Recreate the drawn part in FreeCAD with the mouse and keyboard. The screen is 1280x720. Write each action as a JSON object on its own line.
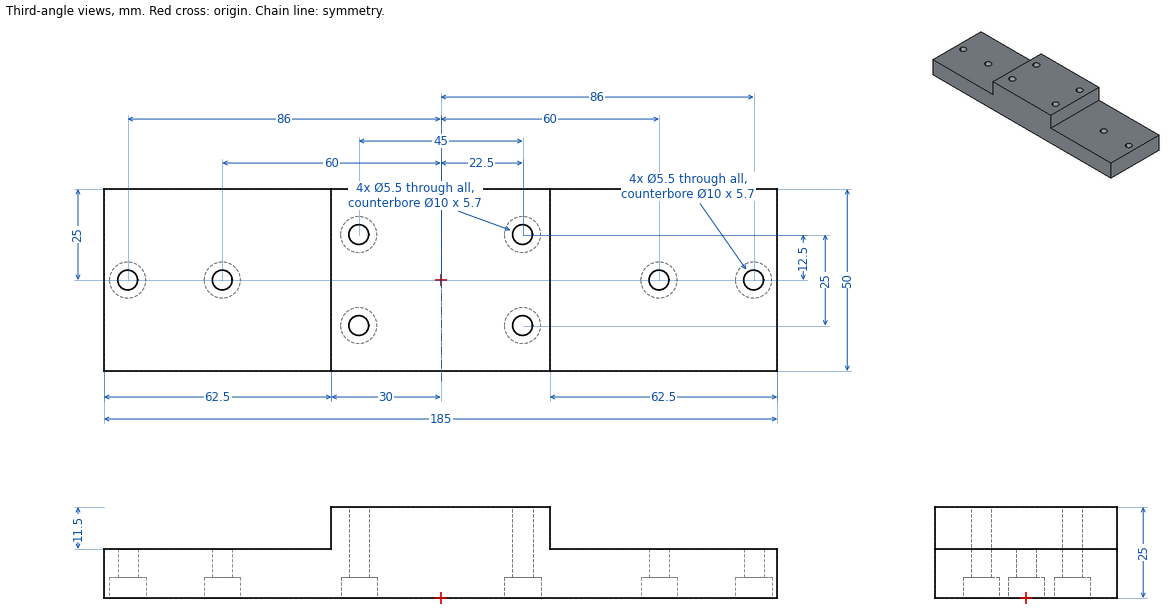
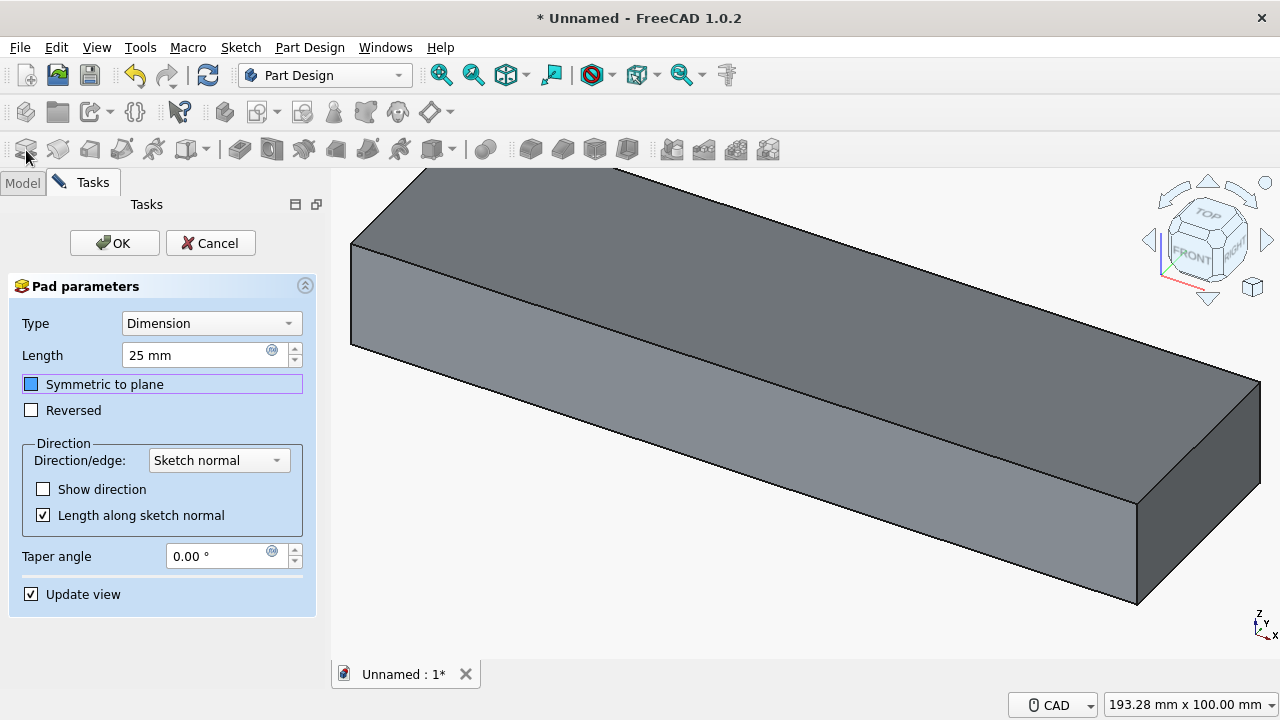
{"action": "left_click", "coordinate": [115, 243]}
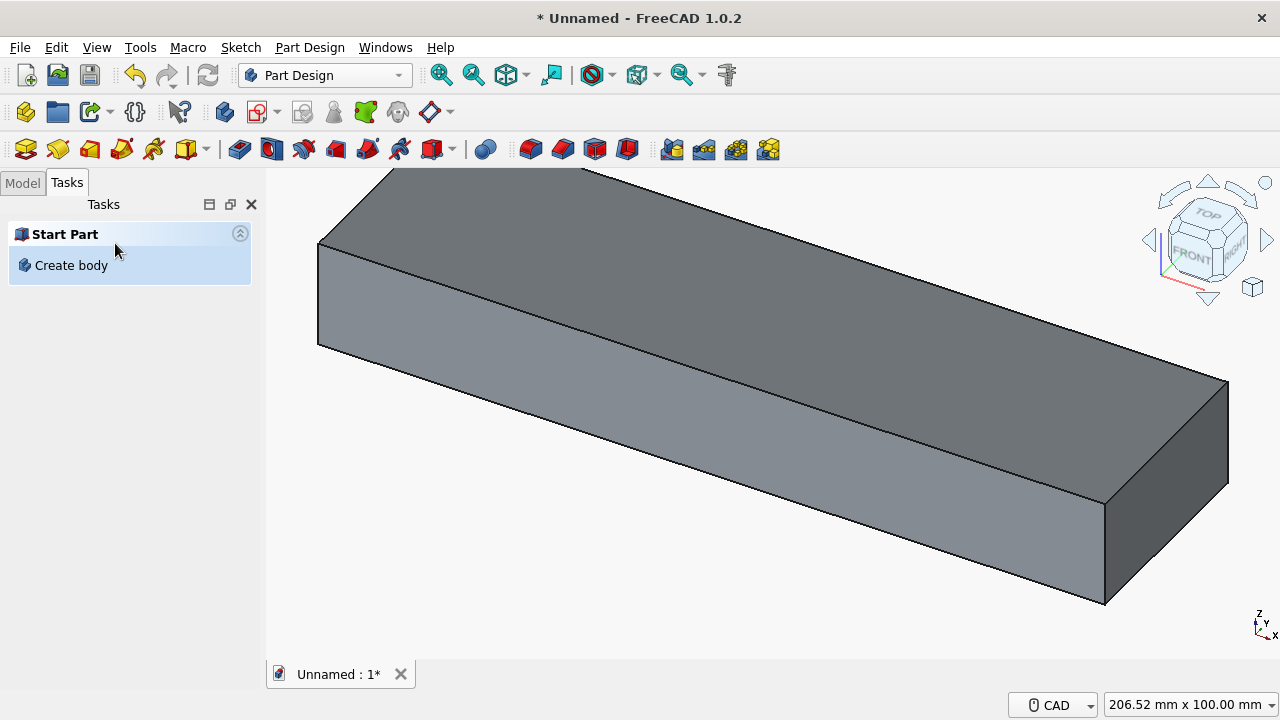
{"action": "key", "text": "v f"}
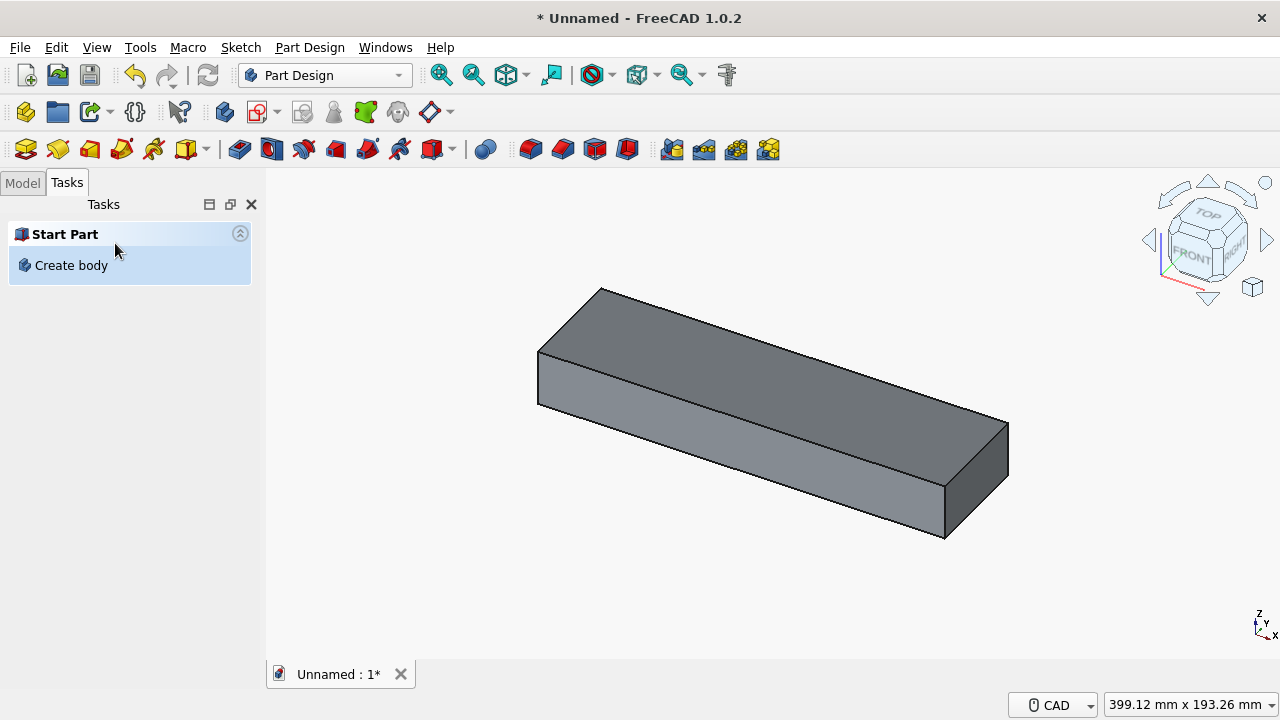
{"action": "left_click", "coordinate": [889, 425]}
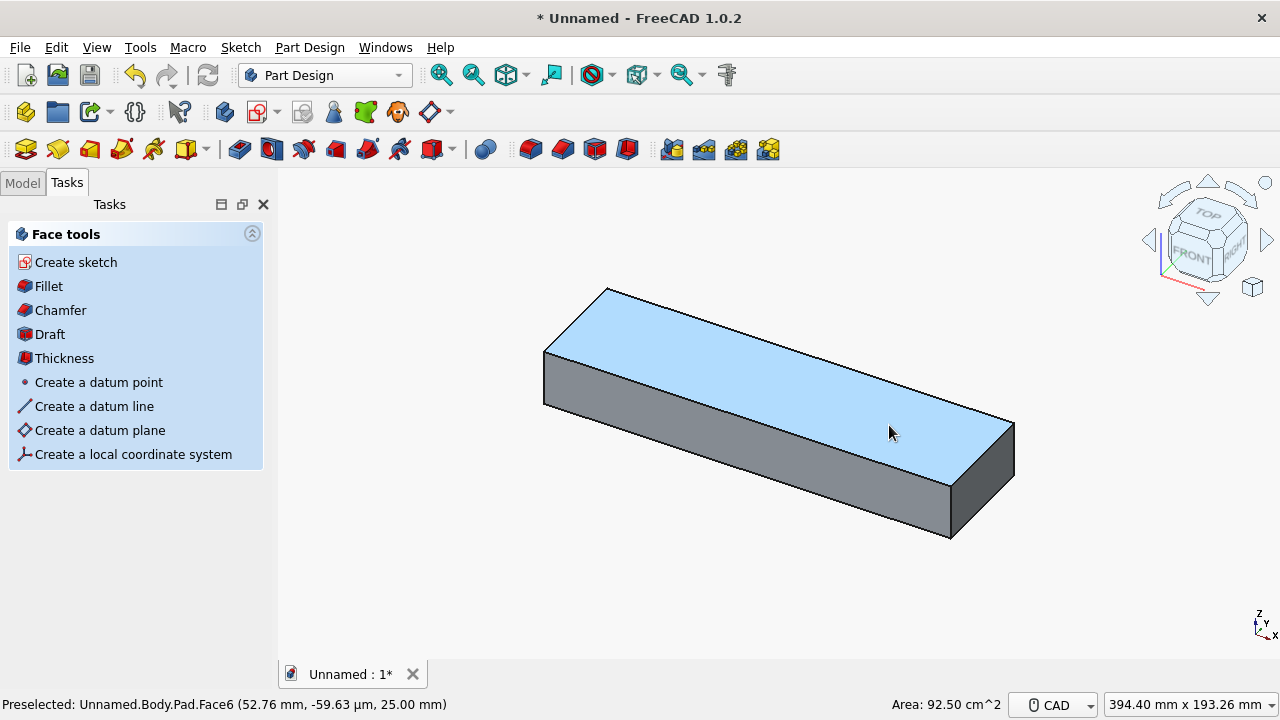
{"action": "left_click", "coordinate": [258, 112]}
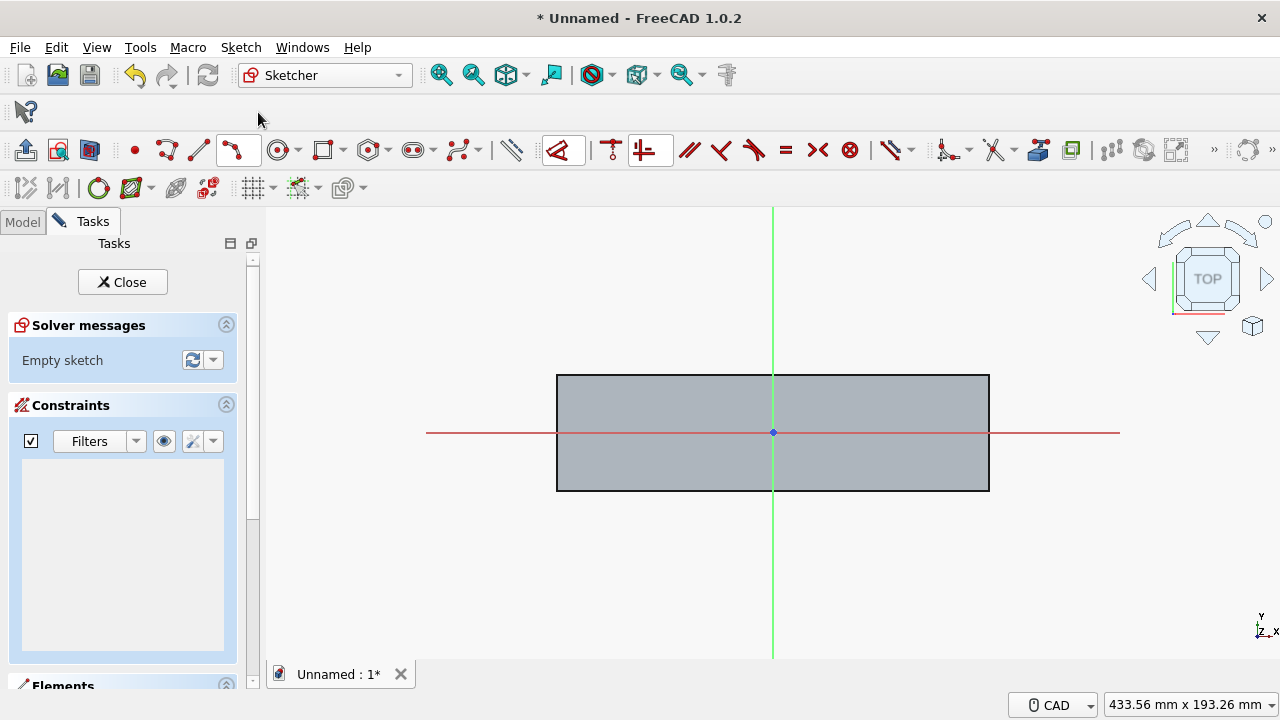
{"action": "key", "text": "g r"}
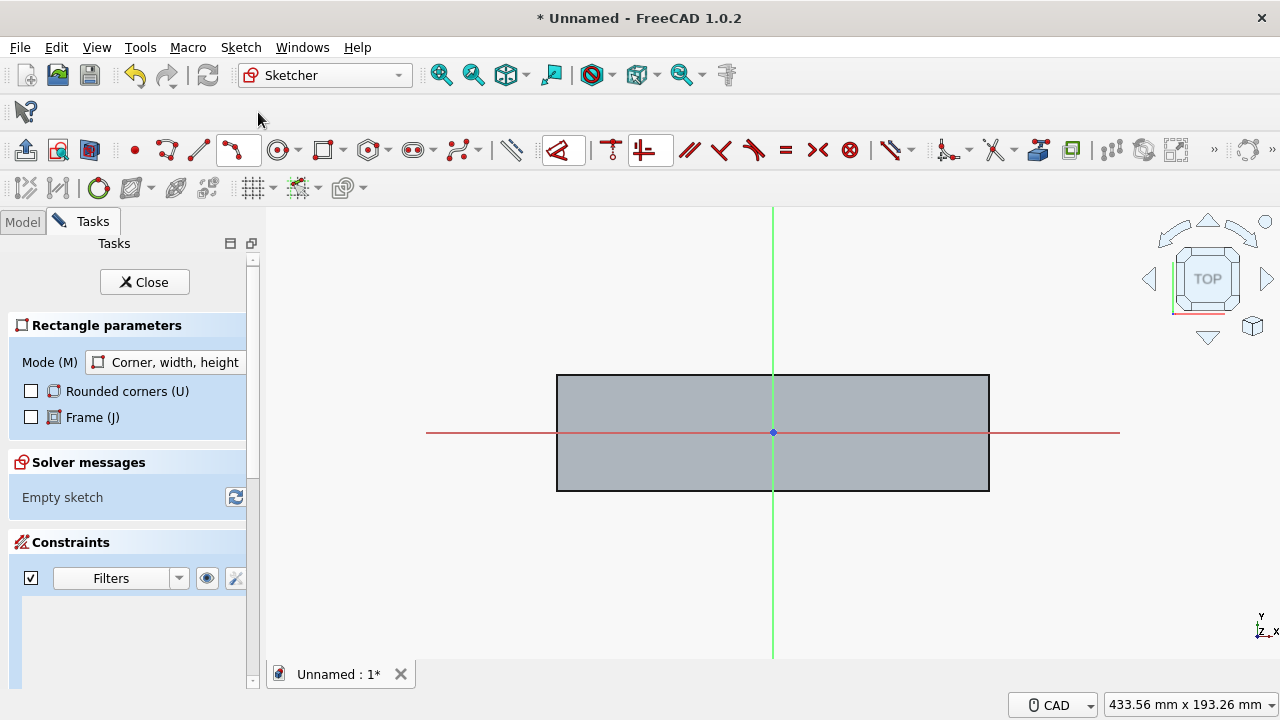
{"action": "left_click", "coordinate": [557, 375]}
{"action": "mouse_move", "coordinate": [703, 491]}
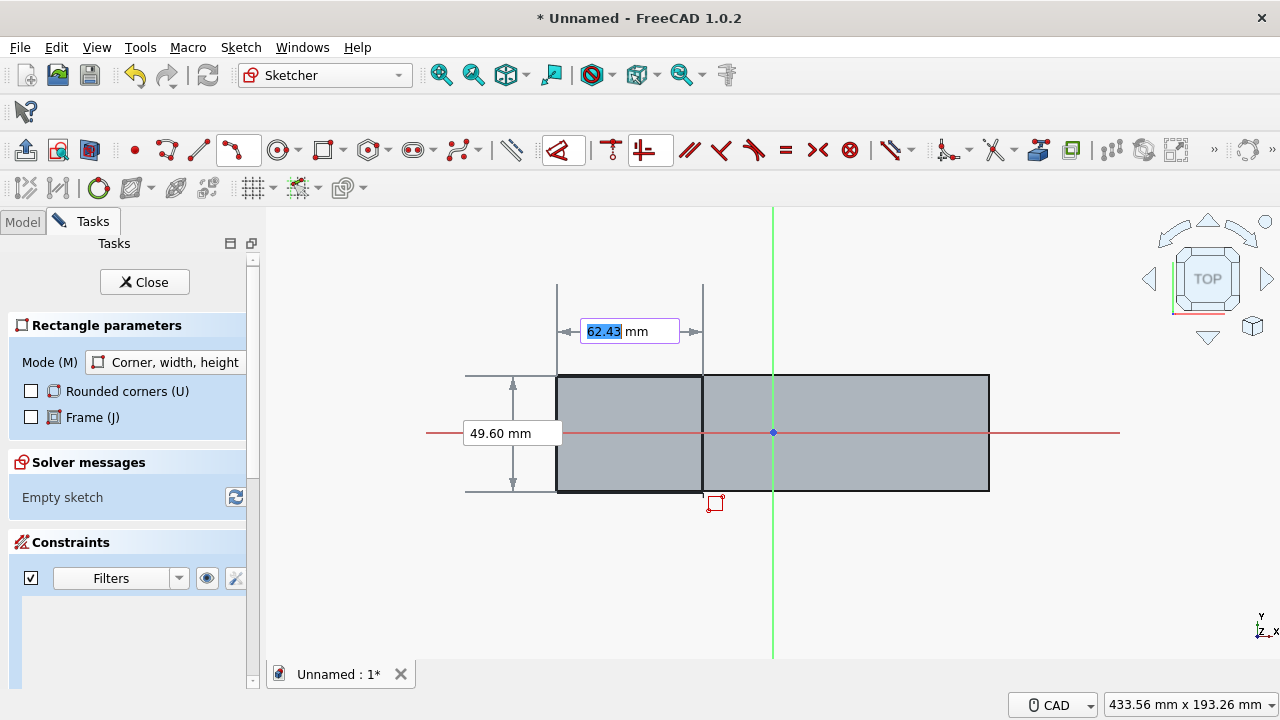
{"action": "type", "text": "62.5"}
{"action": "key", "text": "Tab"}
{"action": "type", "text": "50"}
{"action": "key", "text": "Return"}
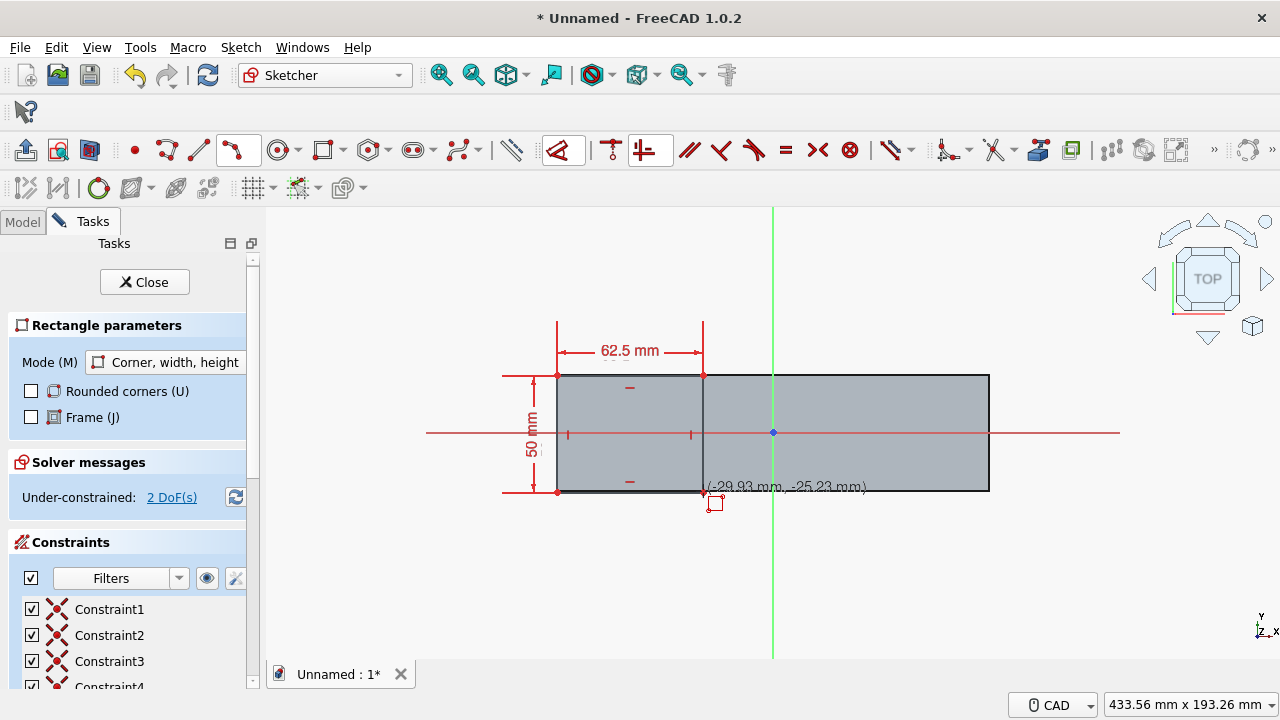
{"action": "left_click", "coordinate": [843, 375]}
{"action": "mouse_move", "coordinate": [989, 491]}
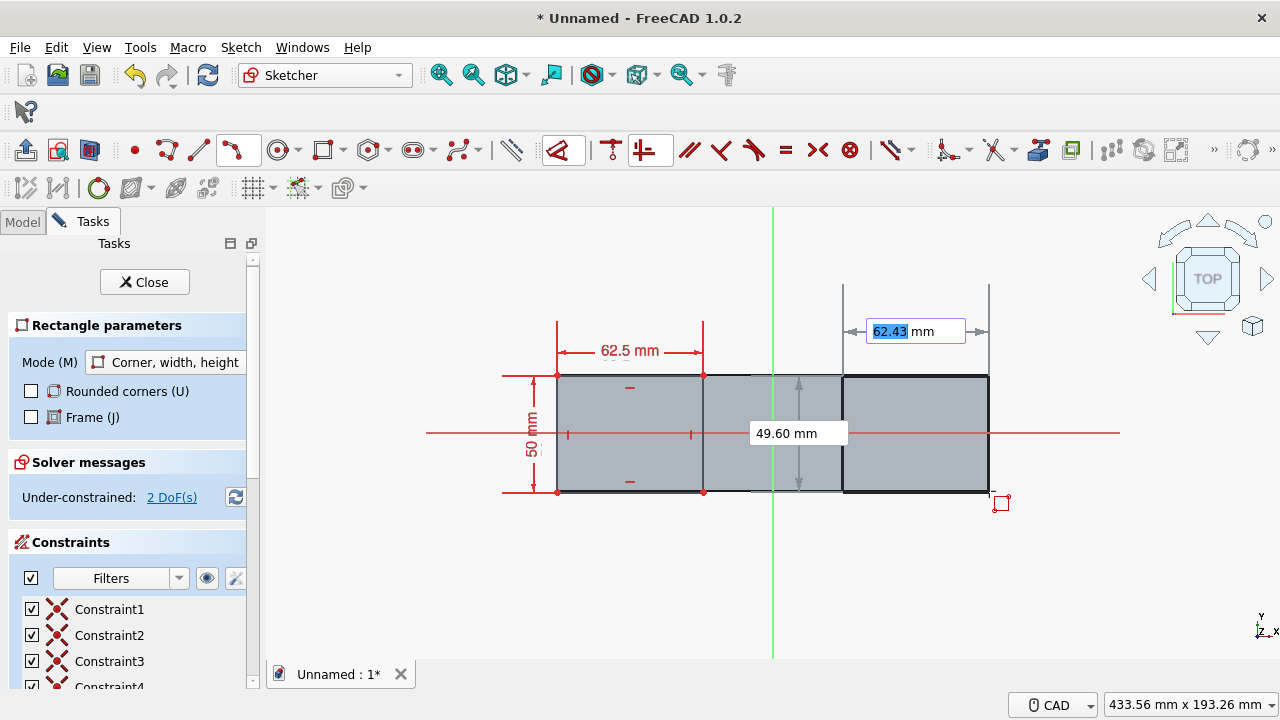
{"action": "type", "text": "62.5"}
{"action": "key", "text": "Tab"}
{"action": "type", "text": "50"}
{"action": "key", "text": "Return"}
{"action": "key", "text": "Escape"}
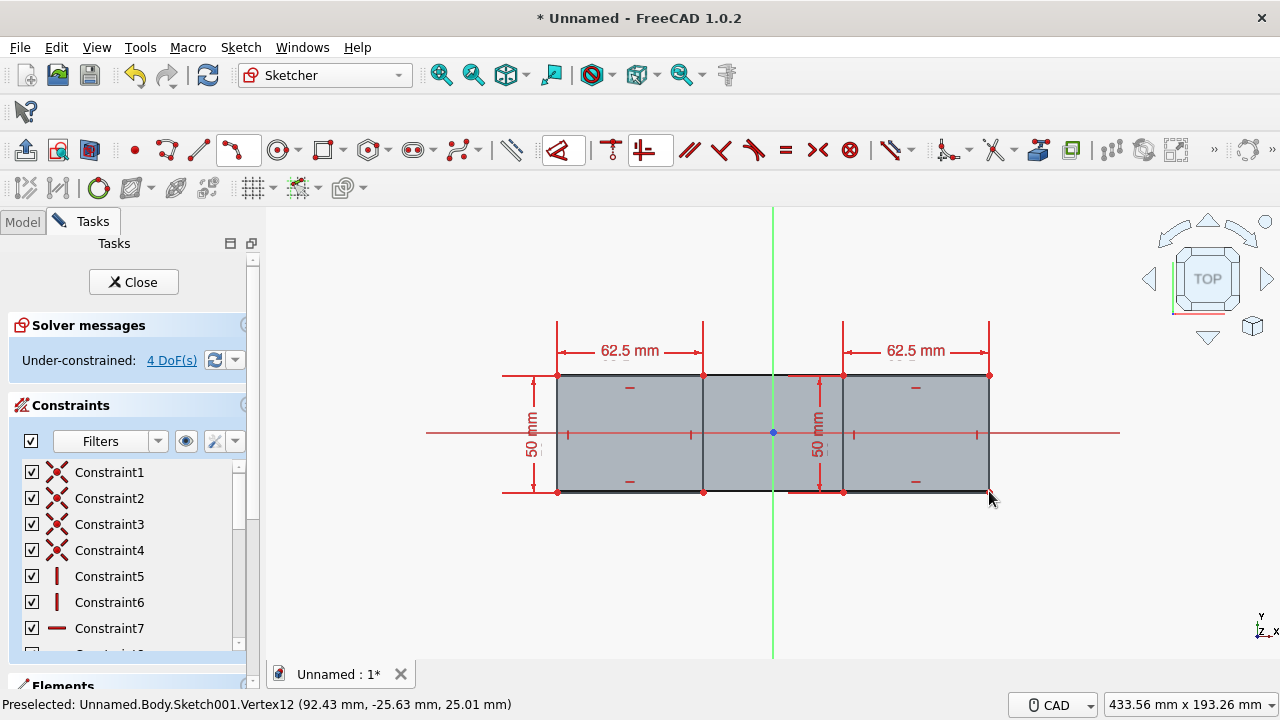
{"action": "left_click", "coordinate": [703, 376]}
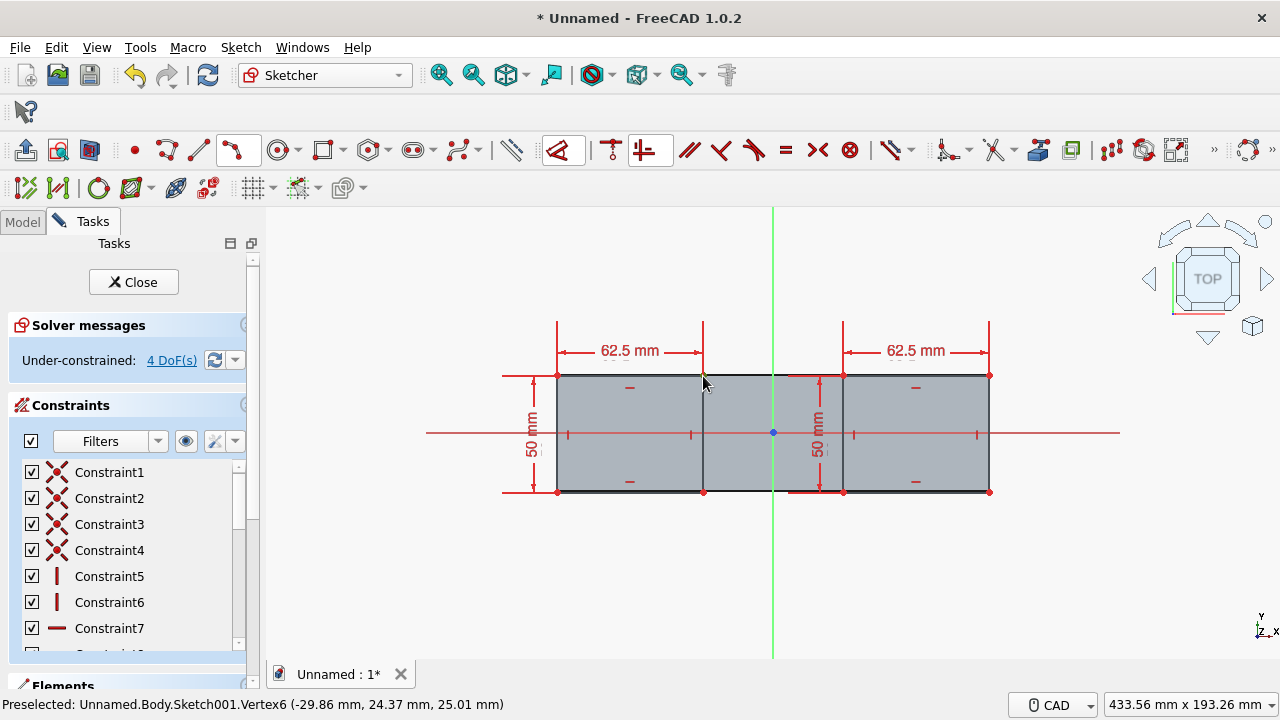
{"action": "left_click", "coordinate": [843, 376]}